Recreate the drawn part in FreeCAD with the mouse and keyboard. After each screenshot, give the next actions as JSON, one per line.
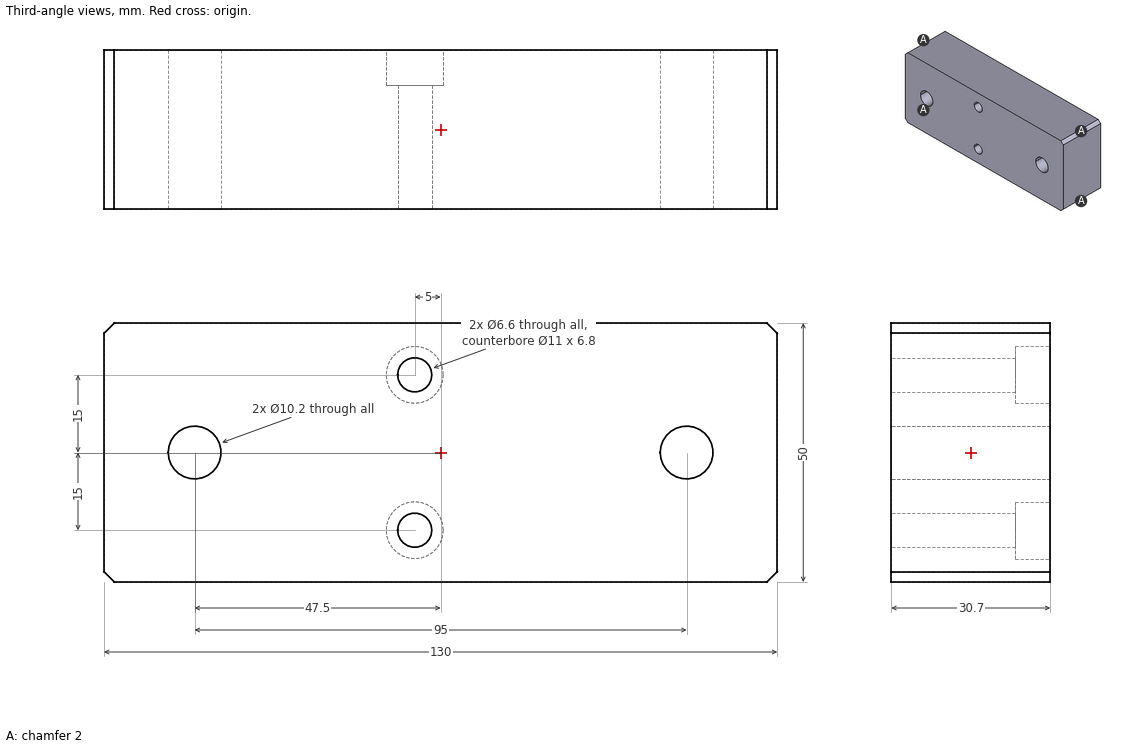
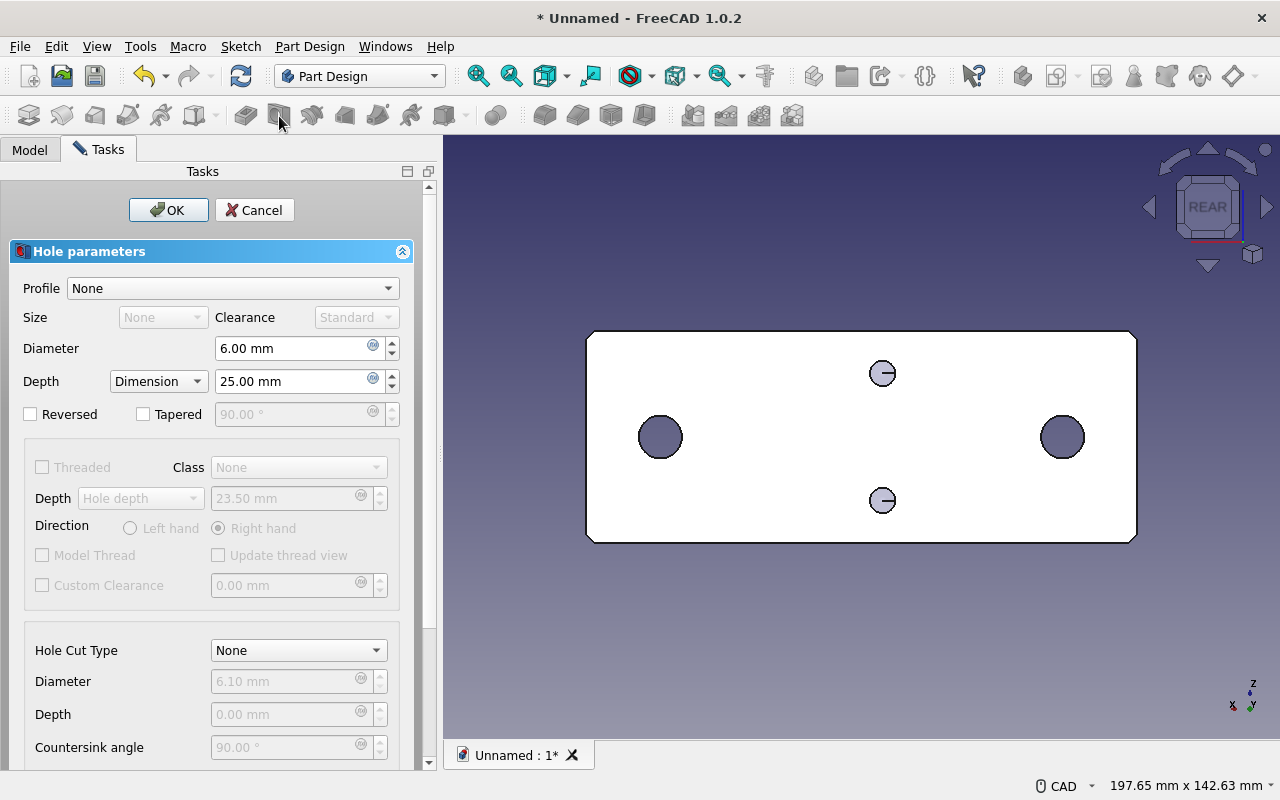
{"action": "triple_click", "coordinate": [300, 348]}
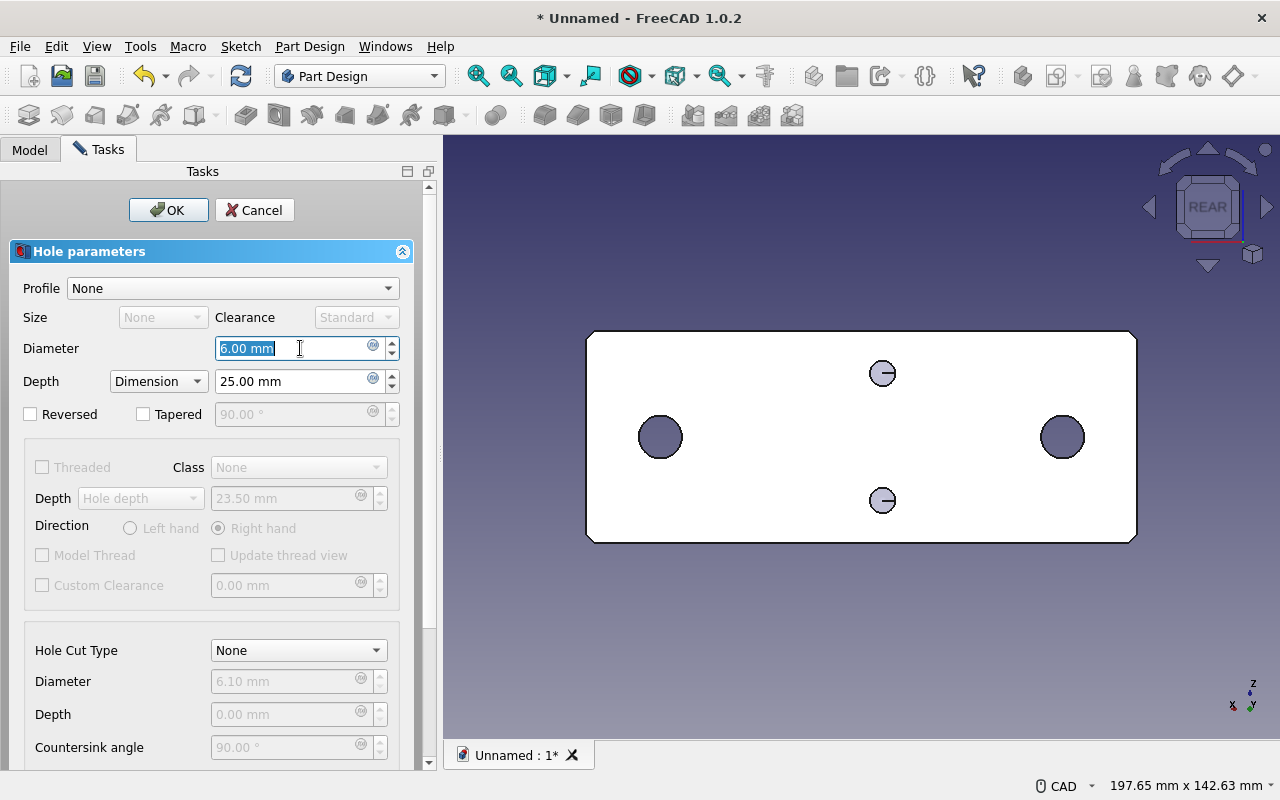
{"action": "type", "text": "6.6"}
{"action": "key", "text": "Tab"}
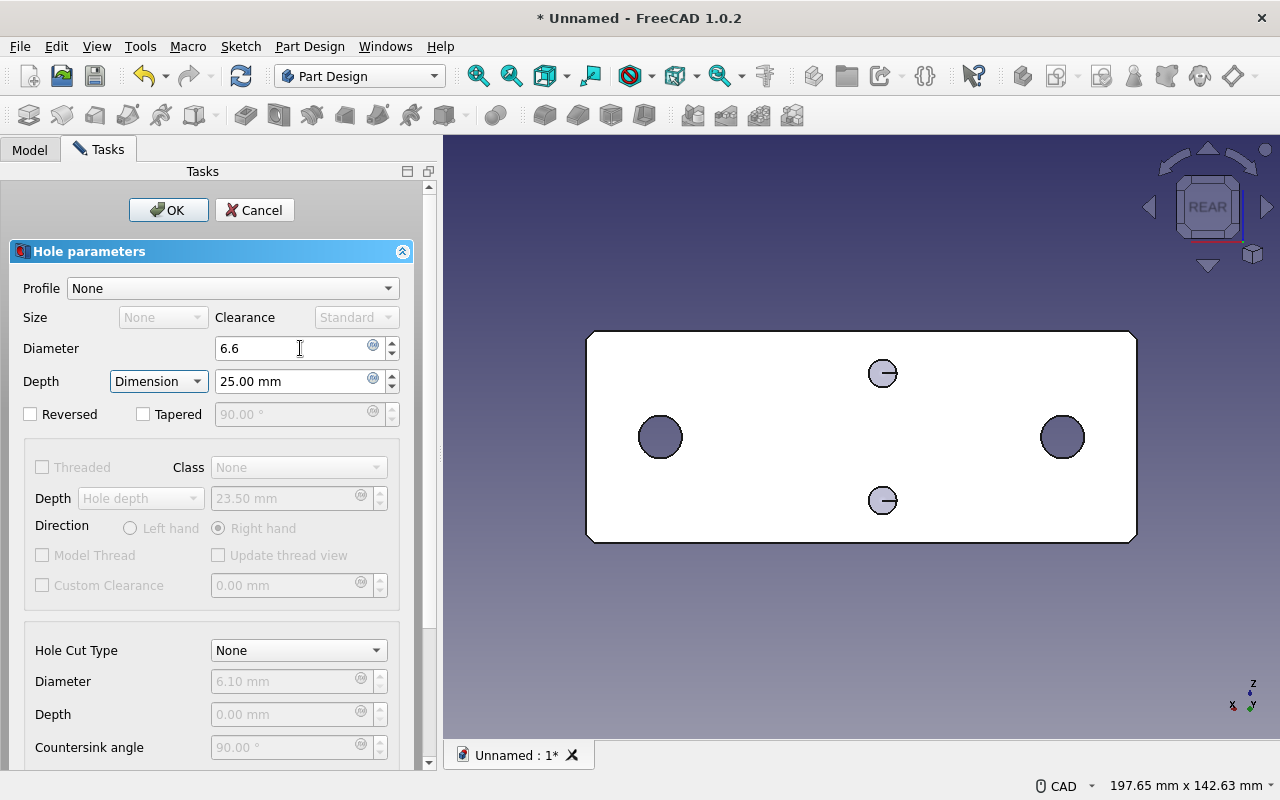
{"action": "left_click", "coordinate": [160, 382]}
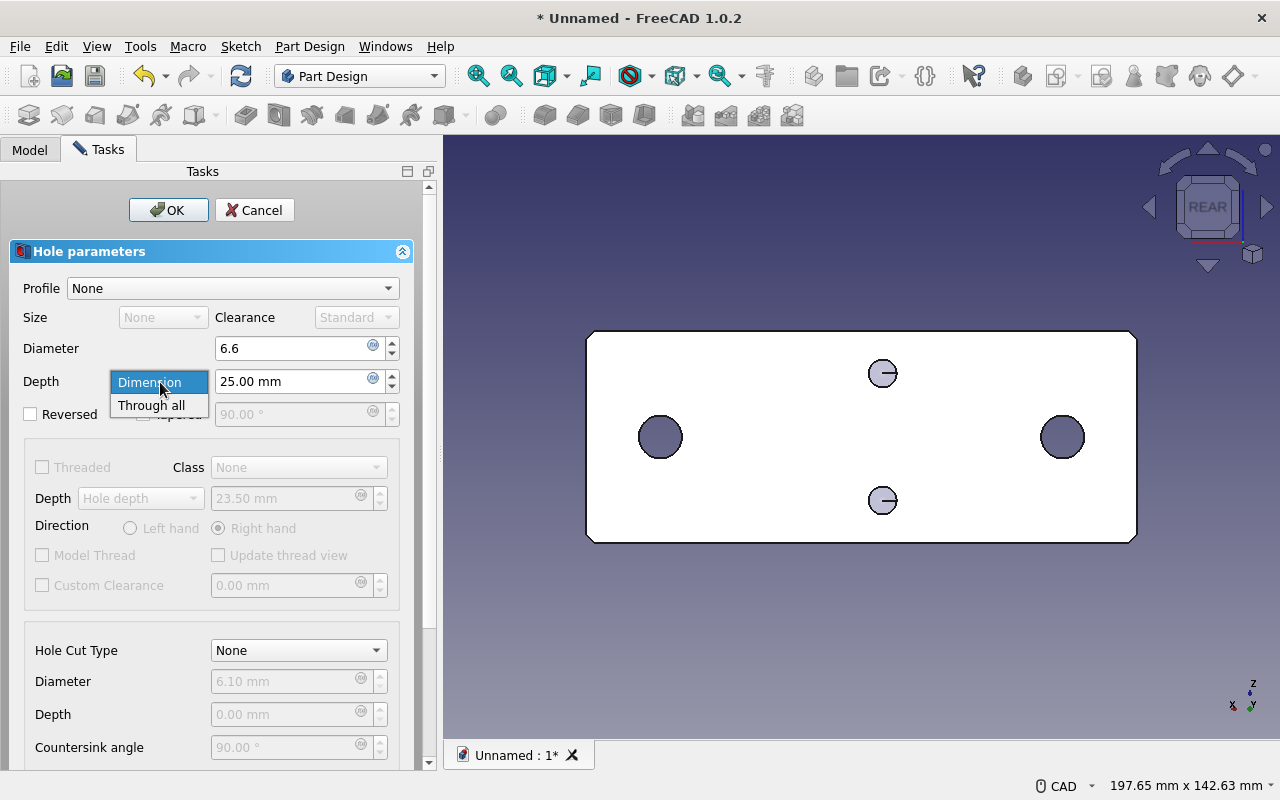
{"action": "left_click", "coordinate": [158, 406]}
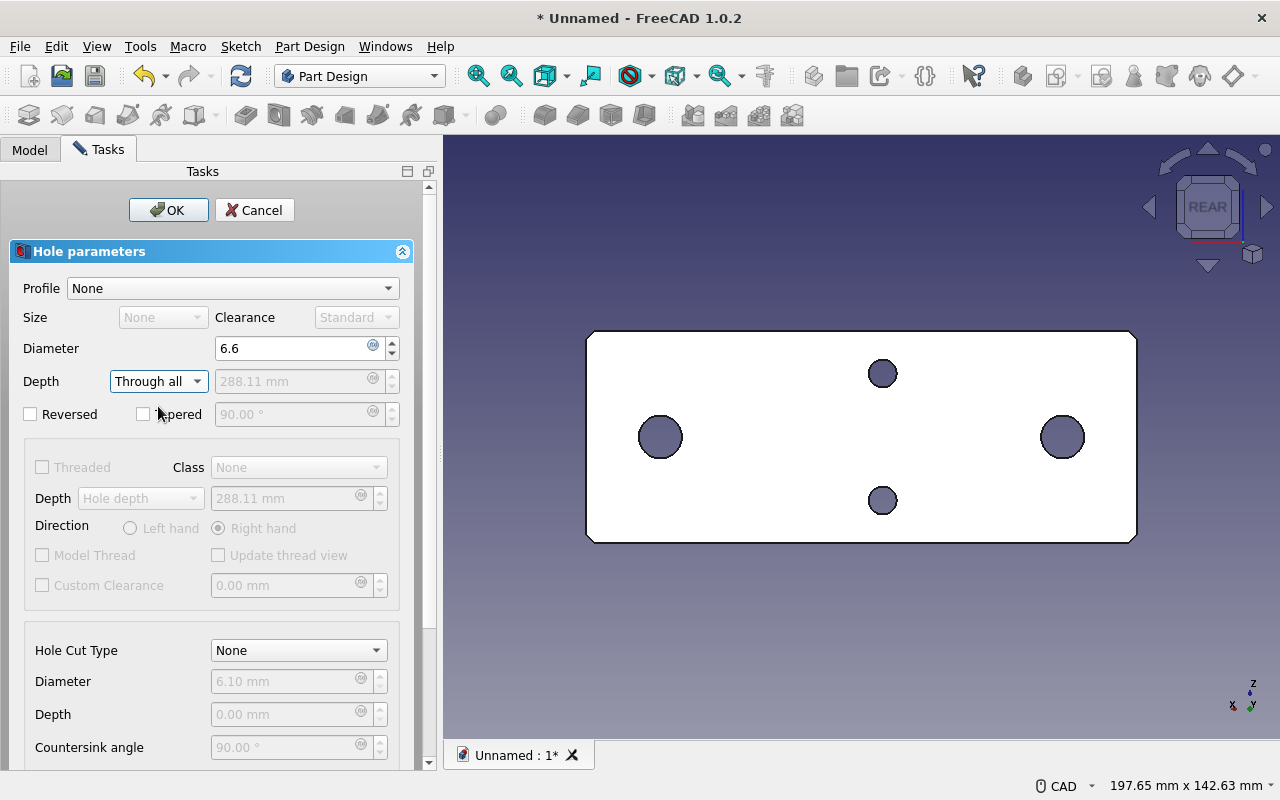
{"action": "left_click", "coordinate": [300, 650]}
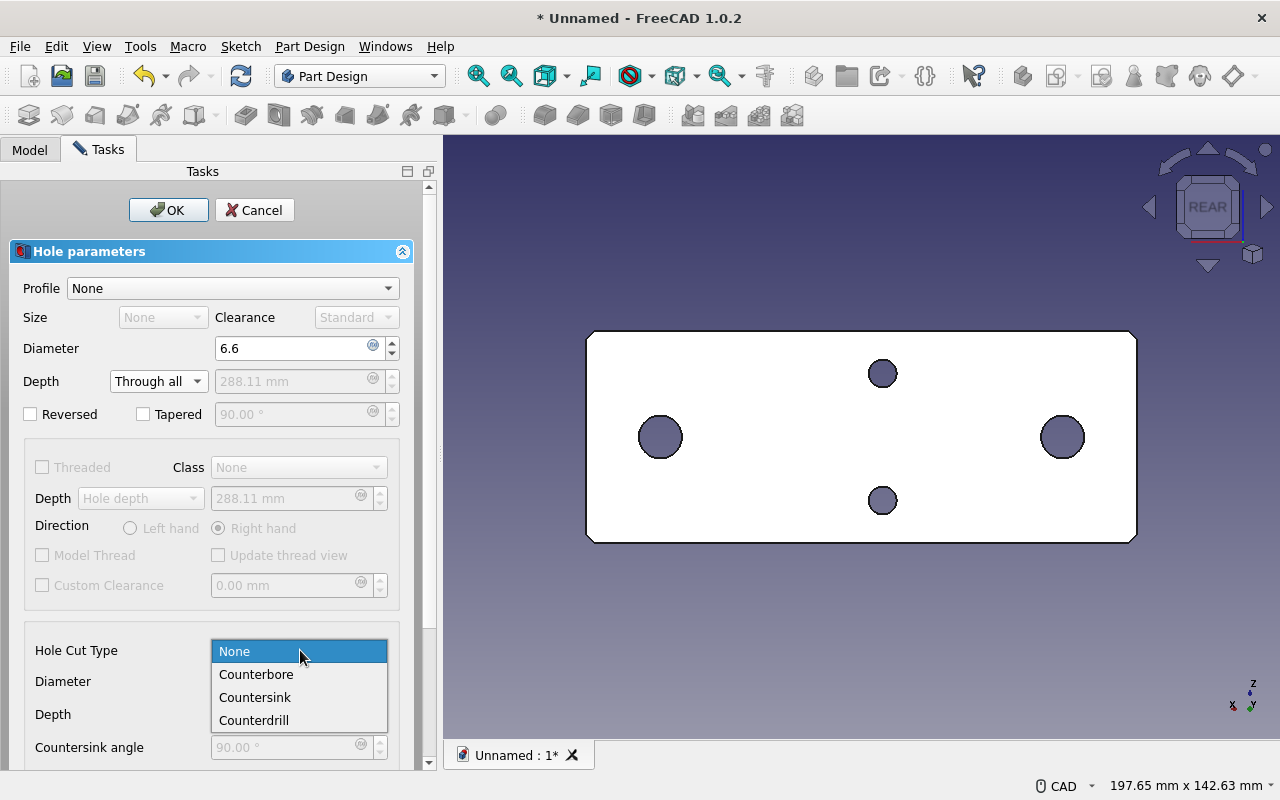
{"action": "left_click", "coordinate": [298, 674]}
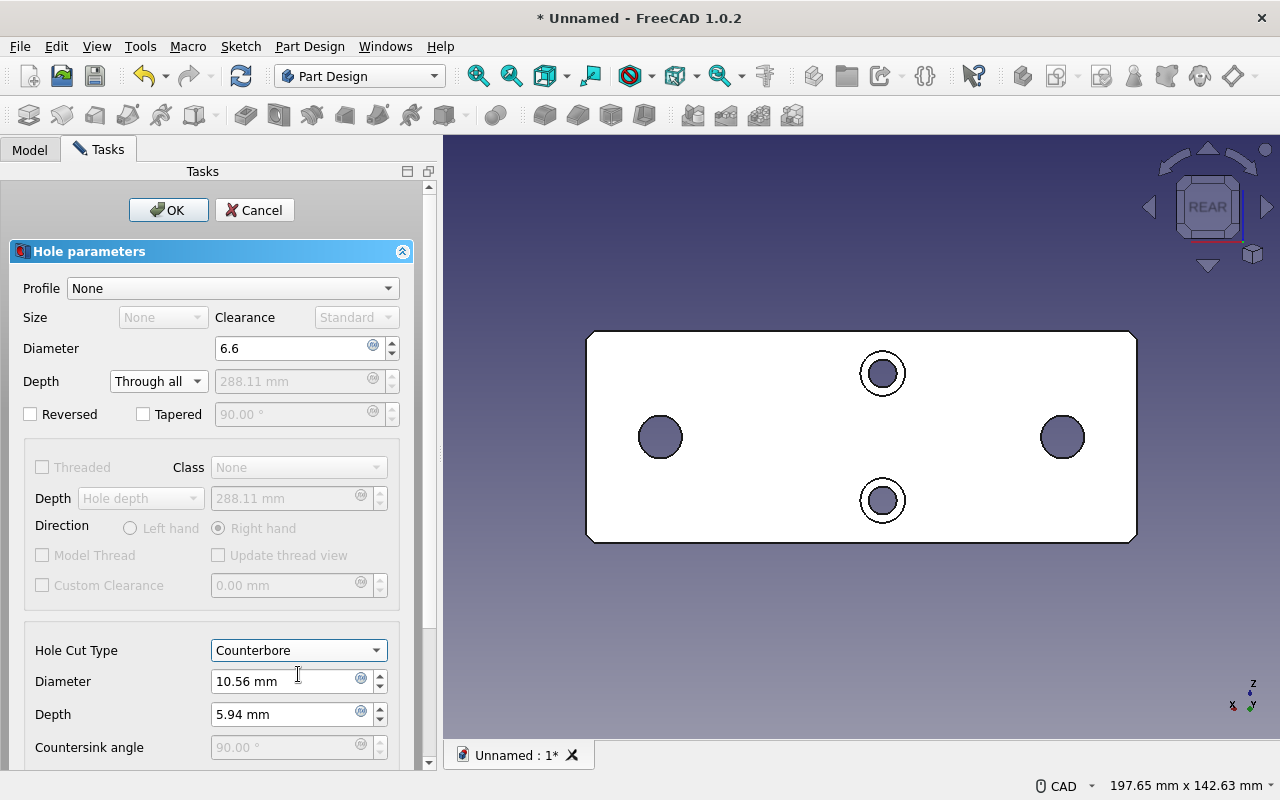
{"action": "triple_click", "coordinate": [292, 682]}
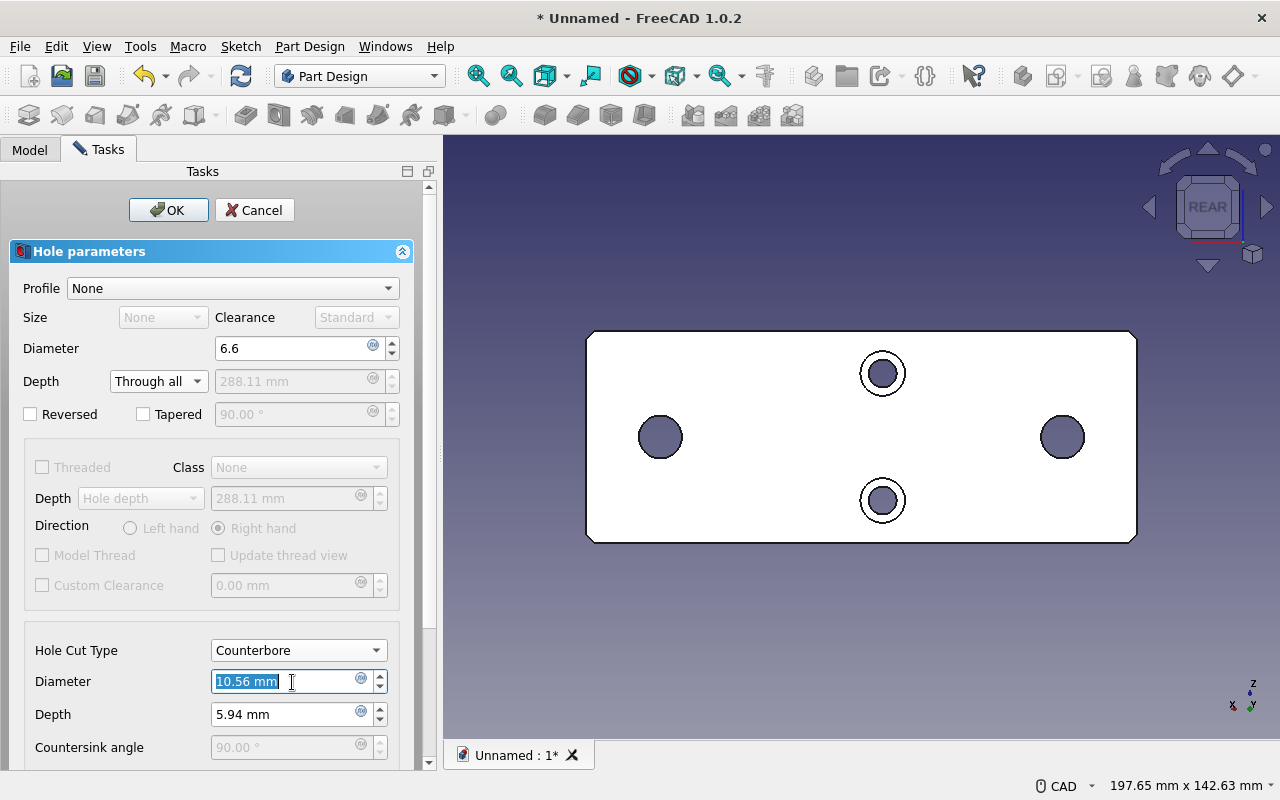
{"action": "type", "text": "11"}
{"action": "key", "text": "Tab"}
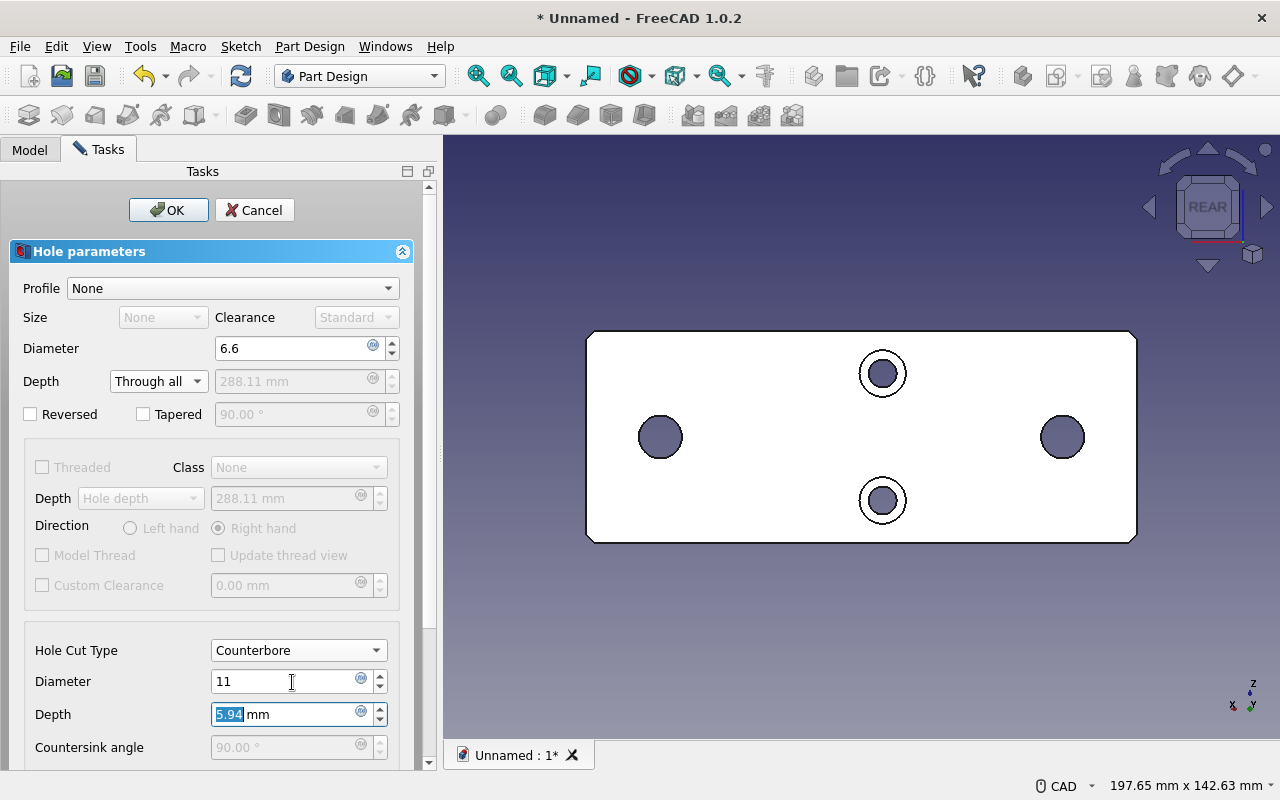
{"action": "type", "text": "6.8"}
{"action": "key", "text": "Tab"}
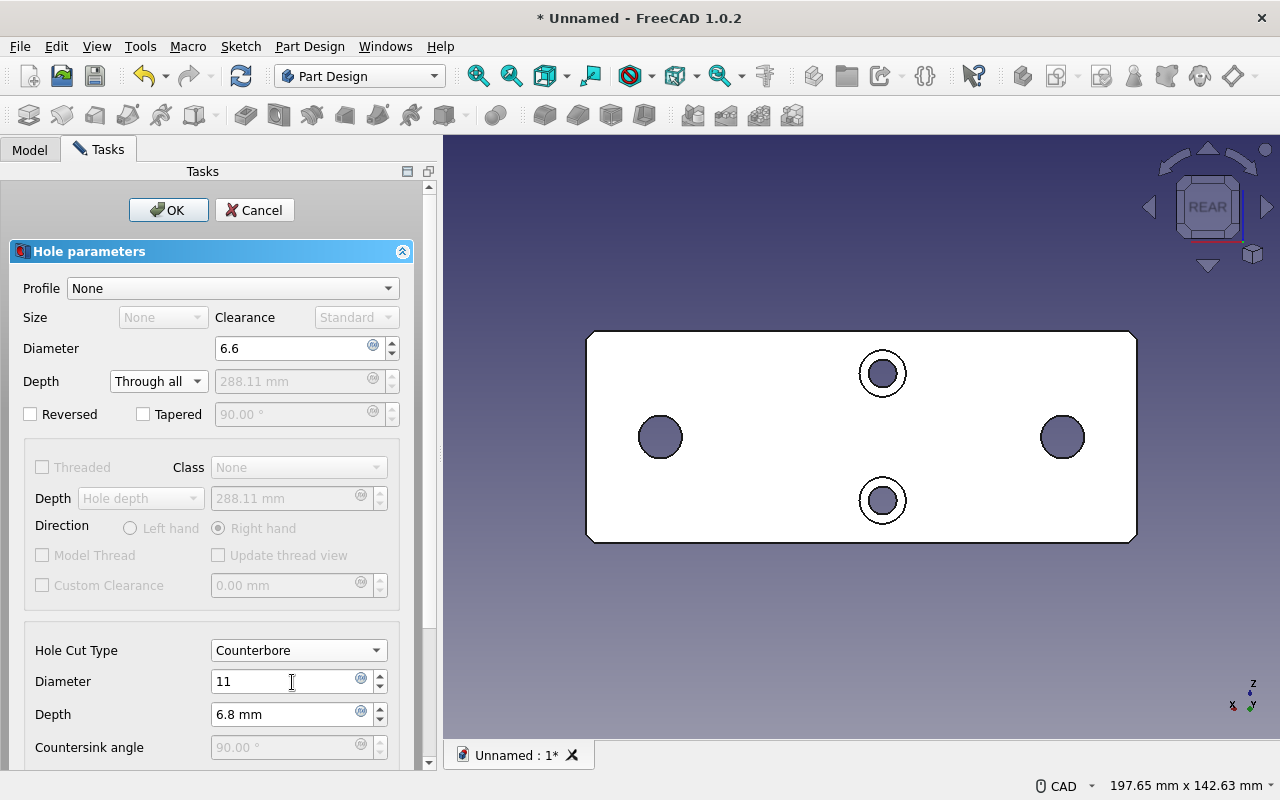
{"action": "left_click", "coordinate": [169, 210]}